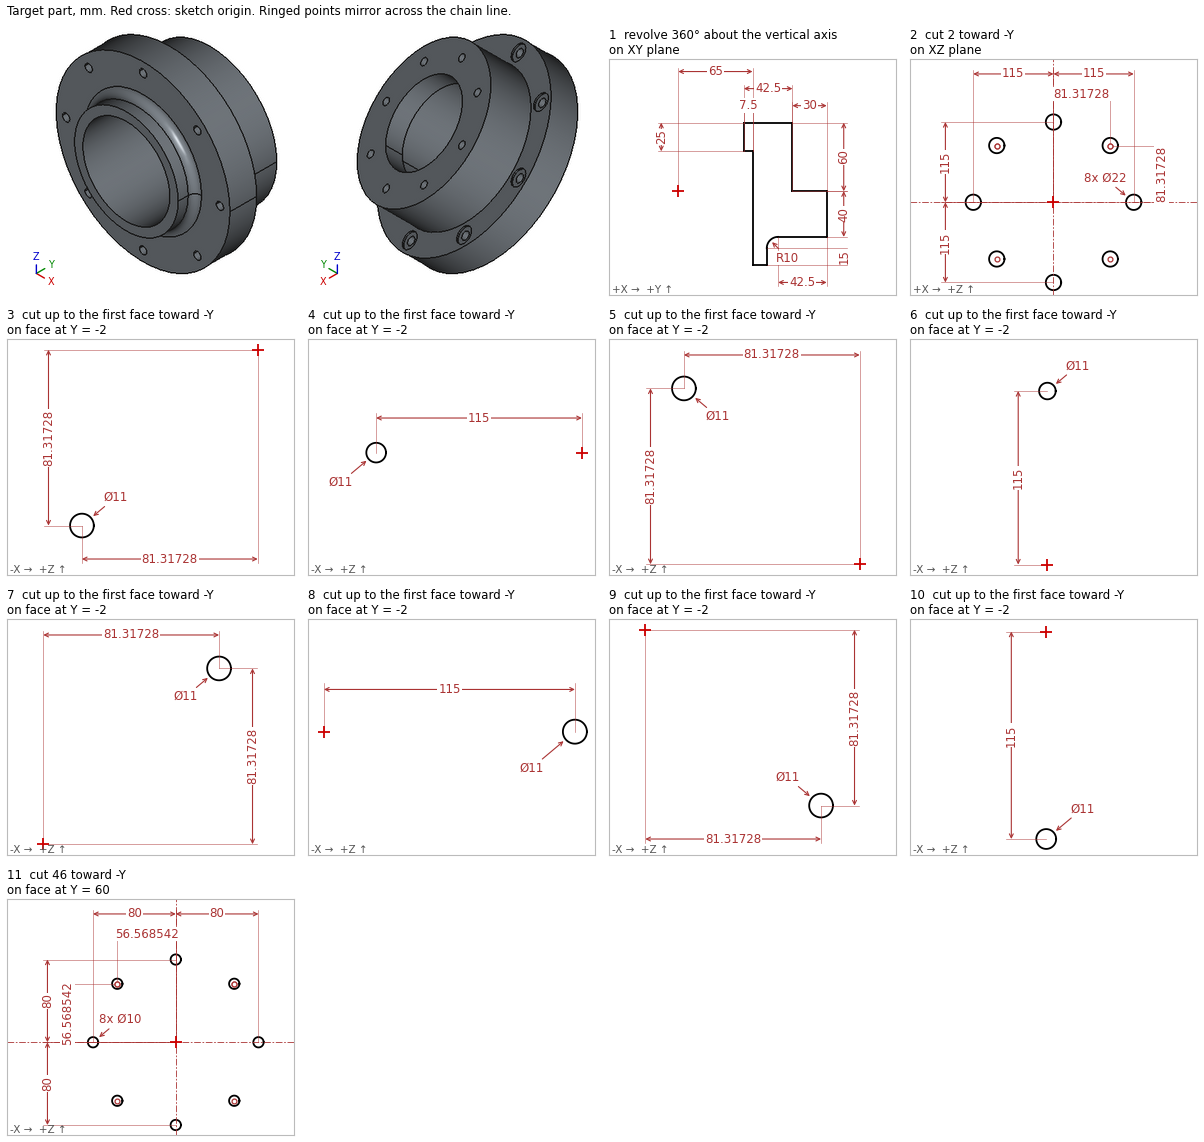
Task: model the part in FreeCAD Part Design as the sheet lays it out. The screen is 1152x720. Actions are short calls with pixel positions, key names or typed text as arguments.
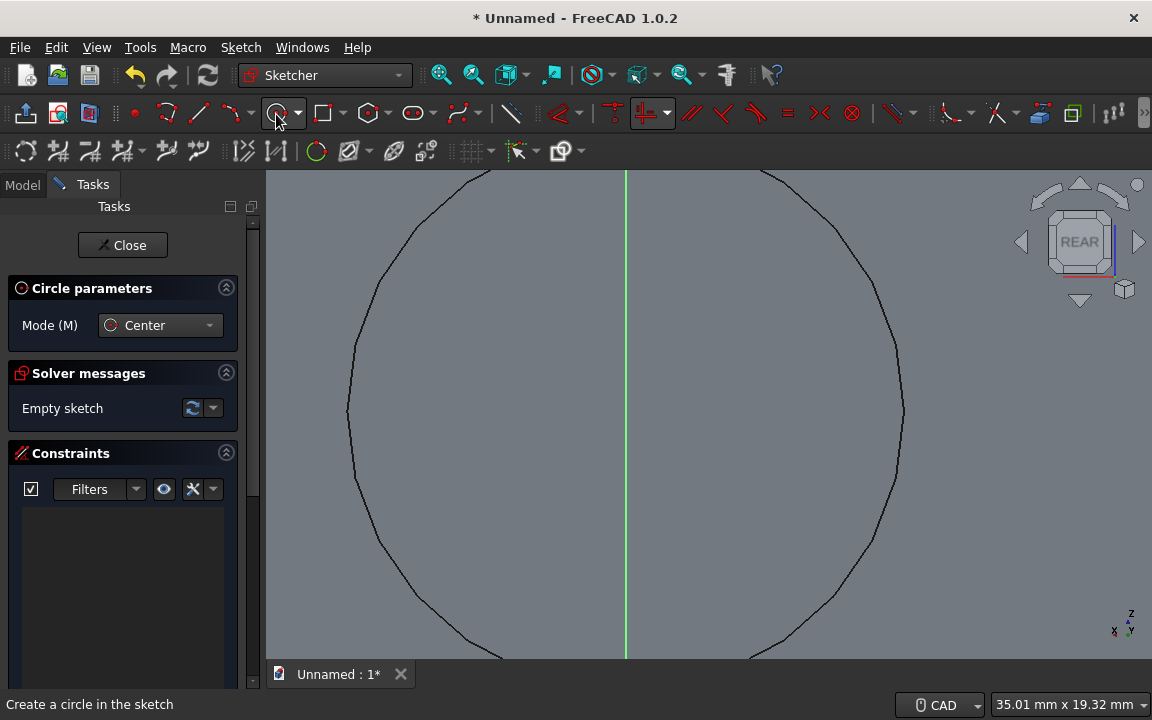
click(626, 411)
move(724, 313)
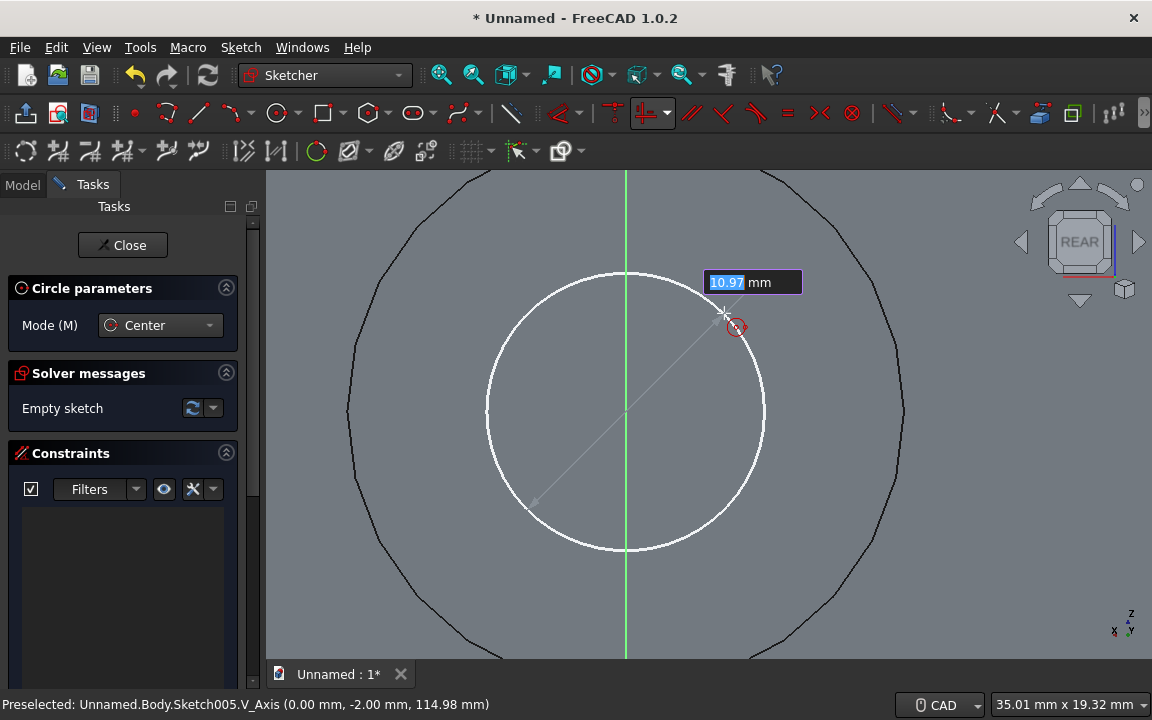
text(11)
key(Return)
key(Escape)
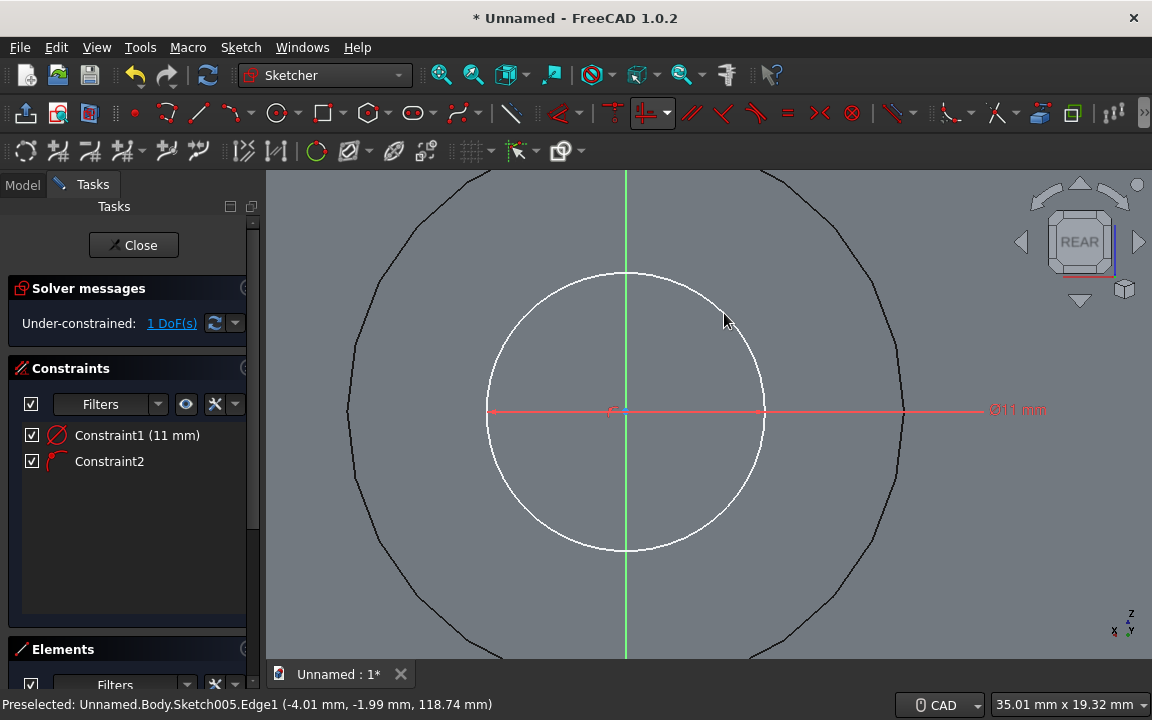
click(558, 114)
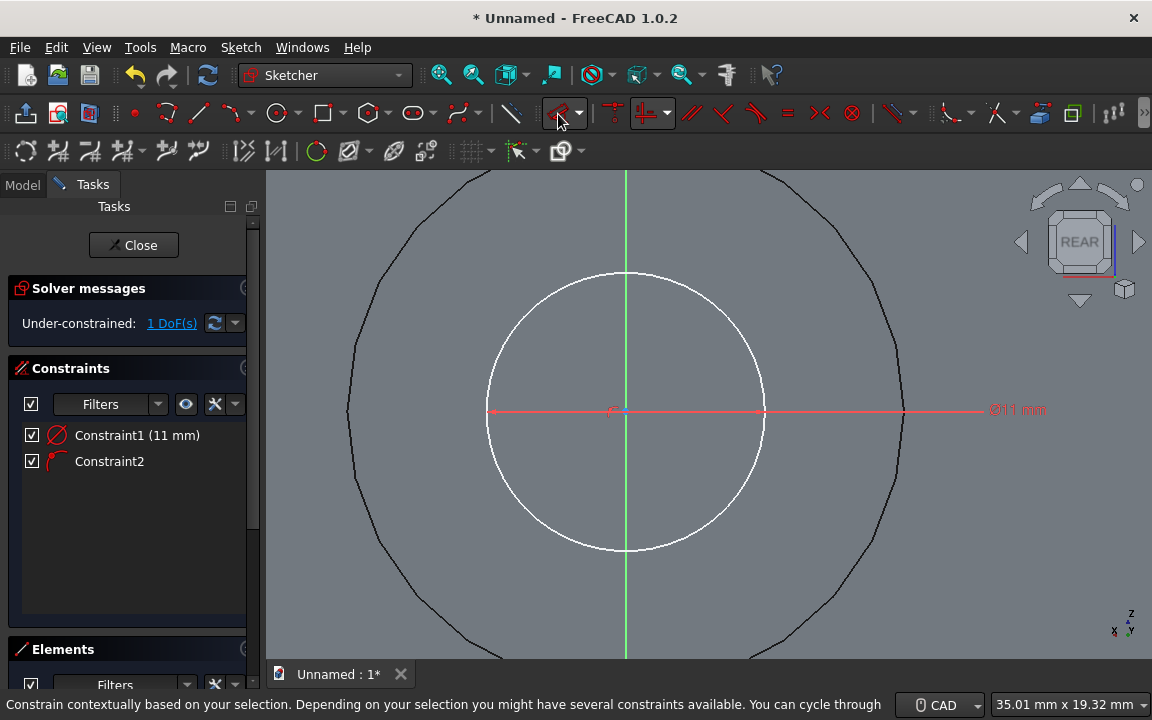
click(626, 412)
click(660, 521)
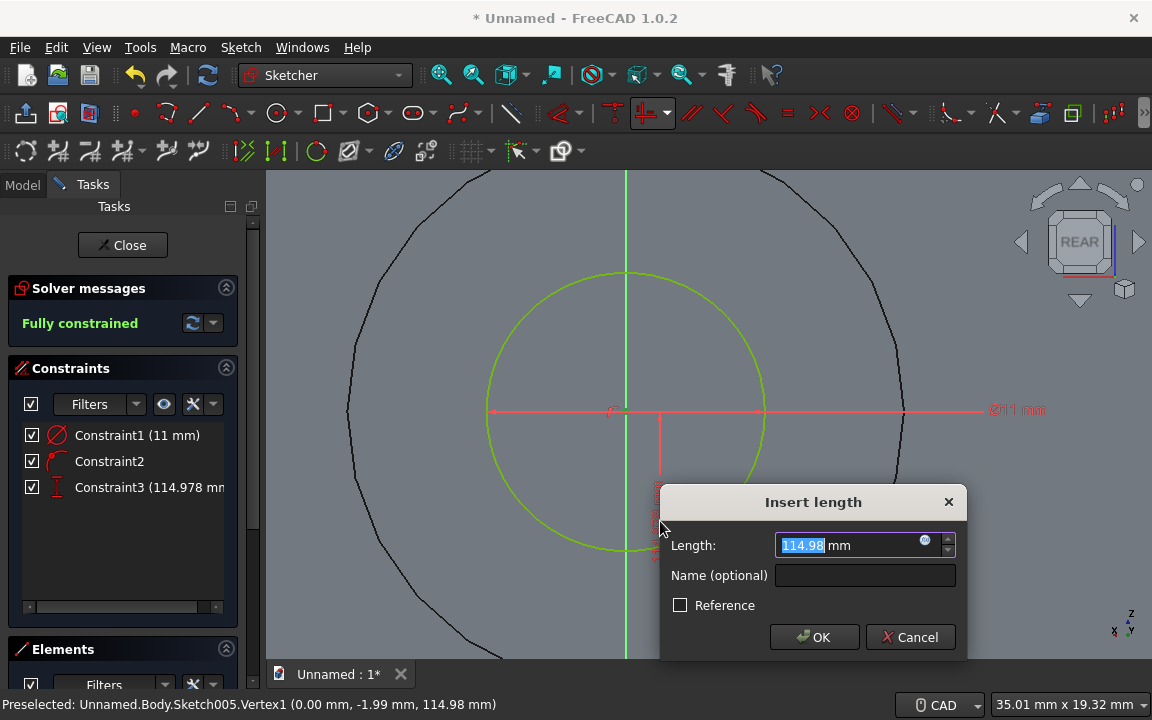
text(115)
key(Return)
key(Escape)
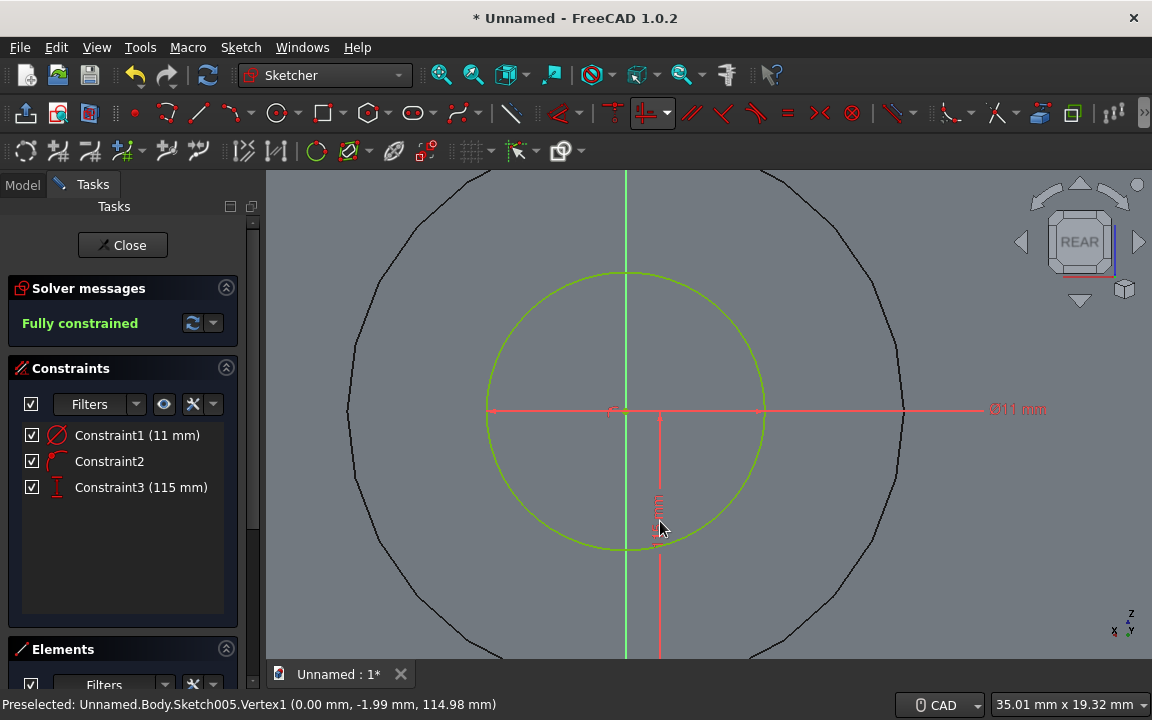
click(123, 245)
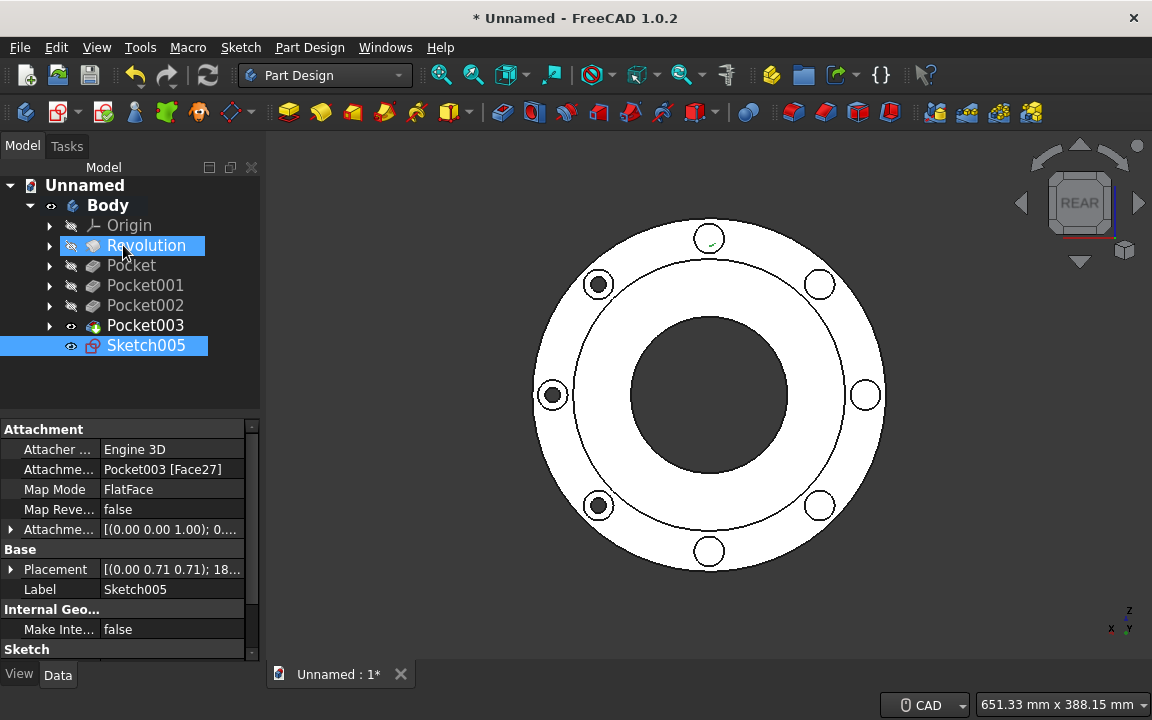
click(504, 112)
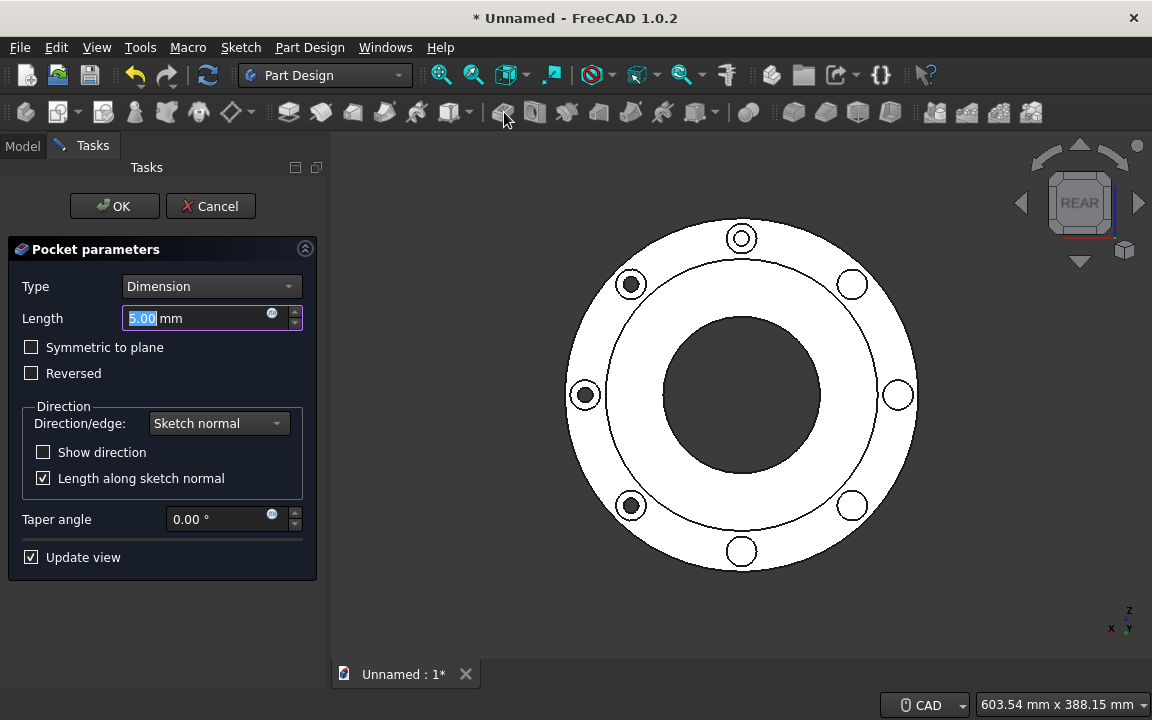
click(212, 286)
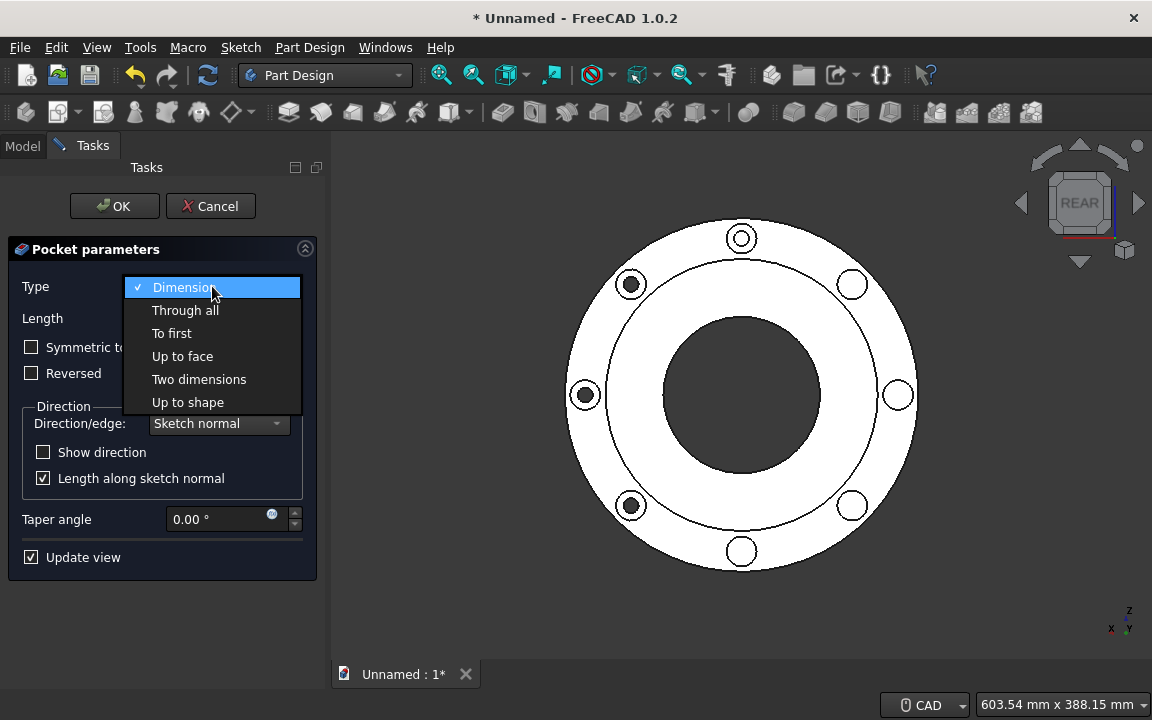
click(212, 334)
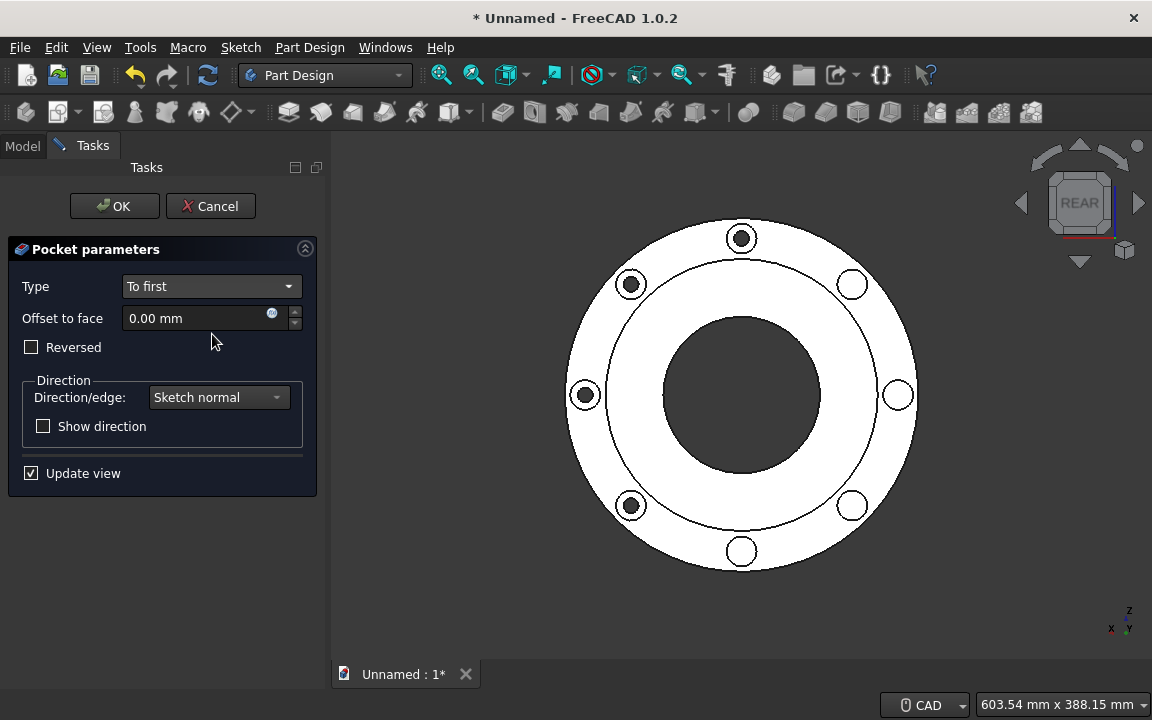
click(115, 206)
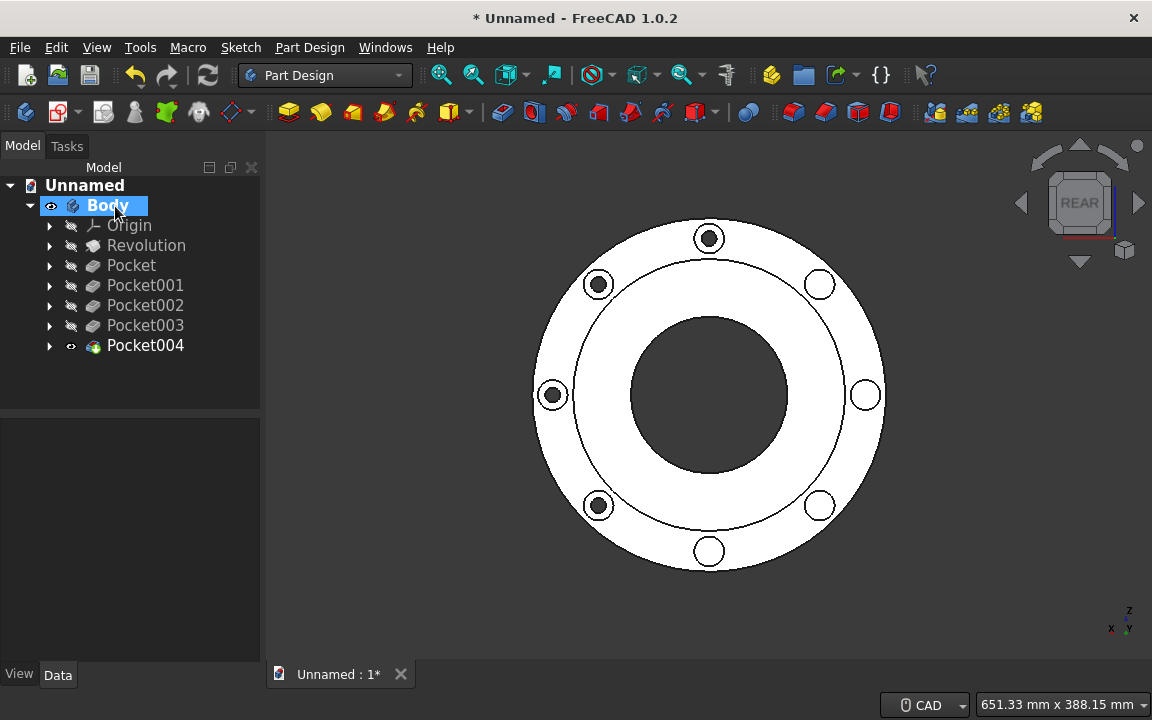
click(820, 283)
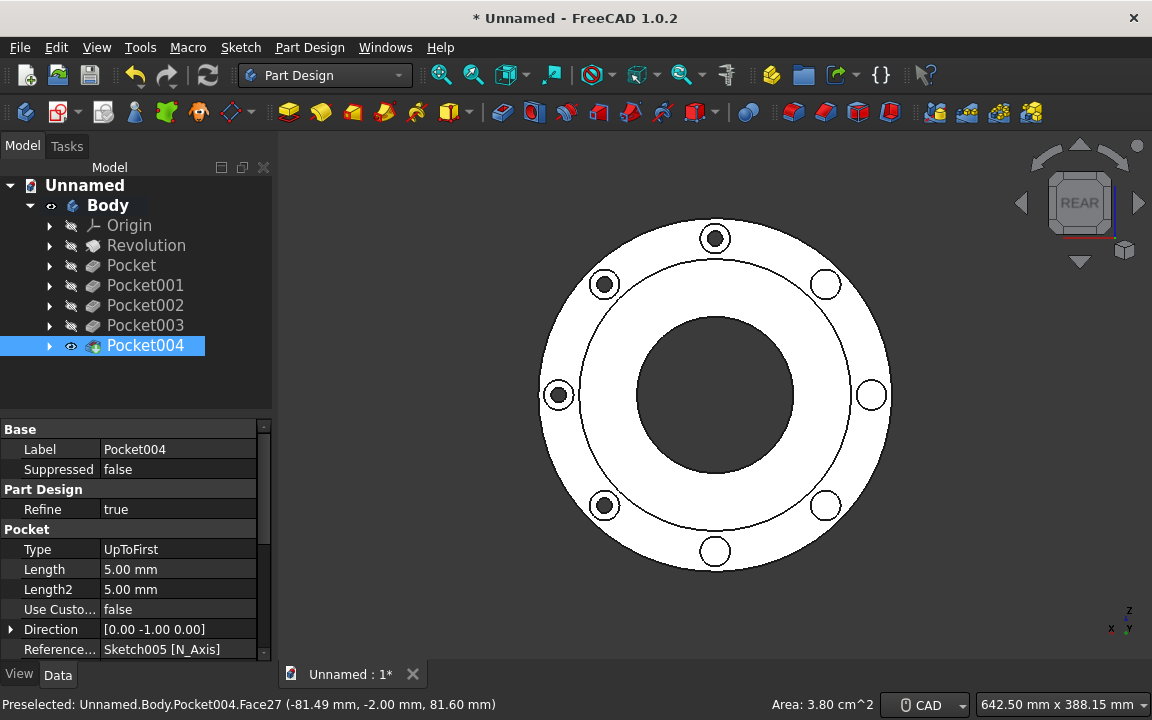
click(58, 112)